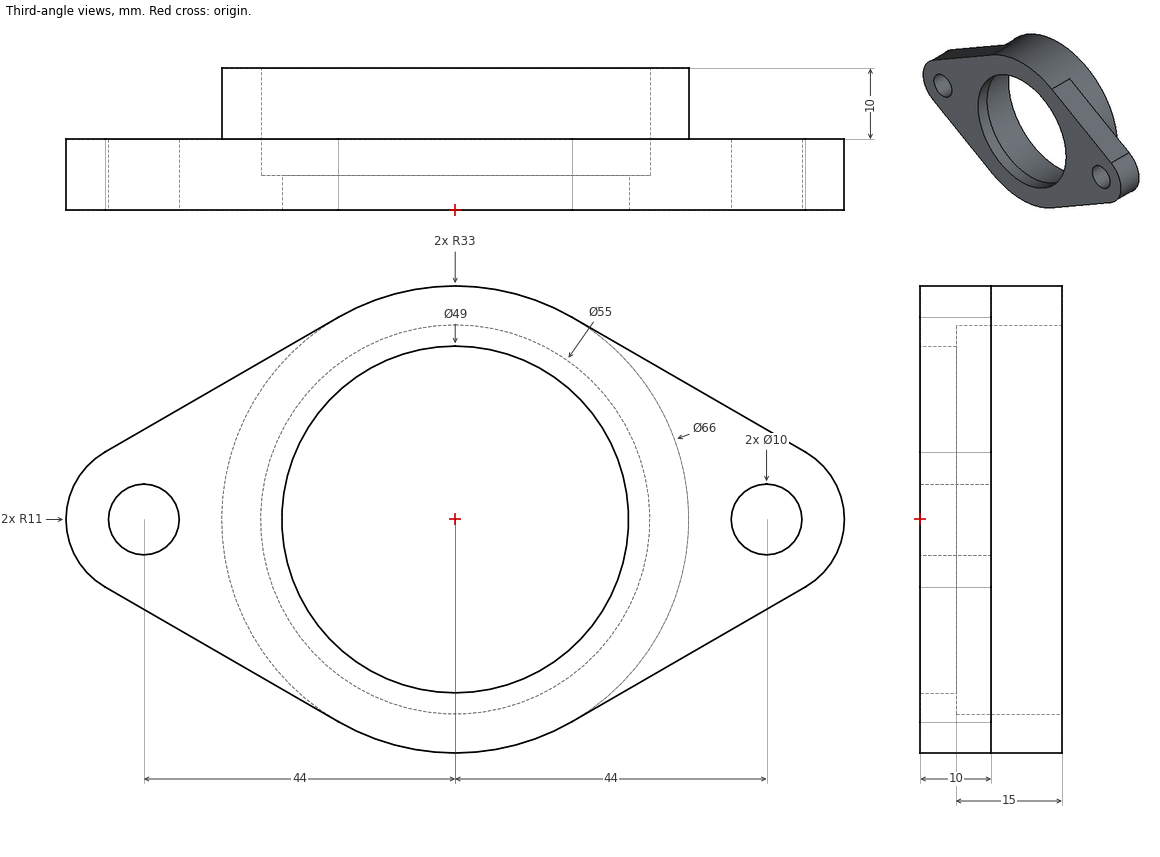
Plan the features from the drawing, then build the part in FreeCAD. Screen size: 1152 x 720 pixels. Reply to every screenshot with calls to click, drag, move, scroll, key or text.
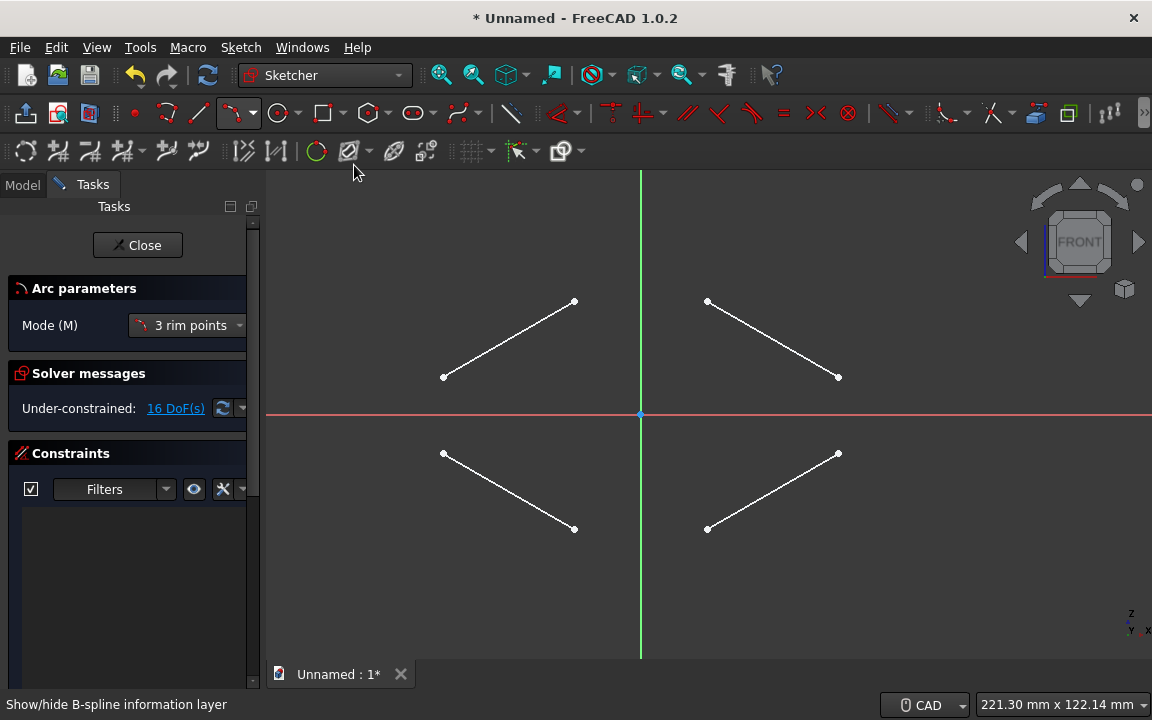
click(443, 454)
click(443, 377)
click(424, 397)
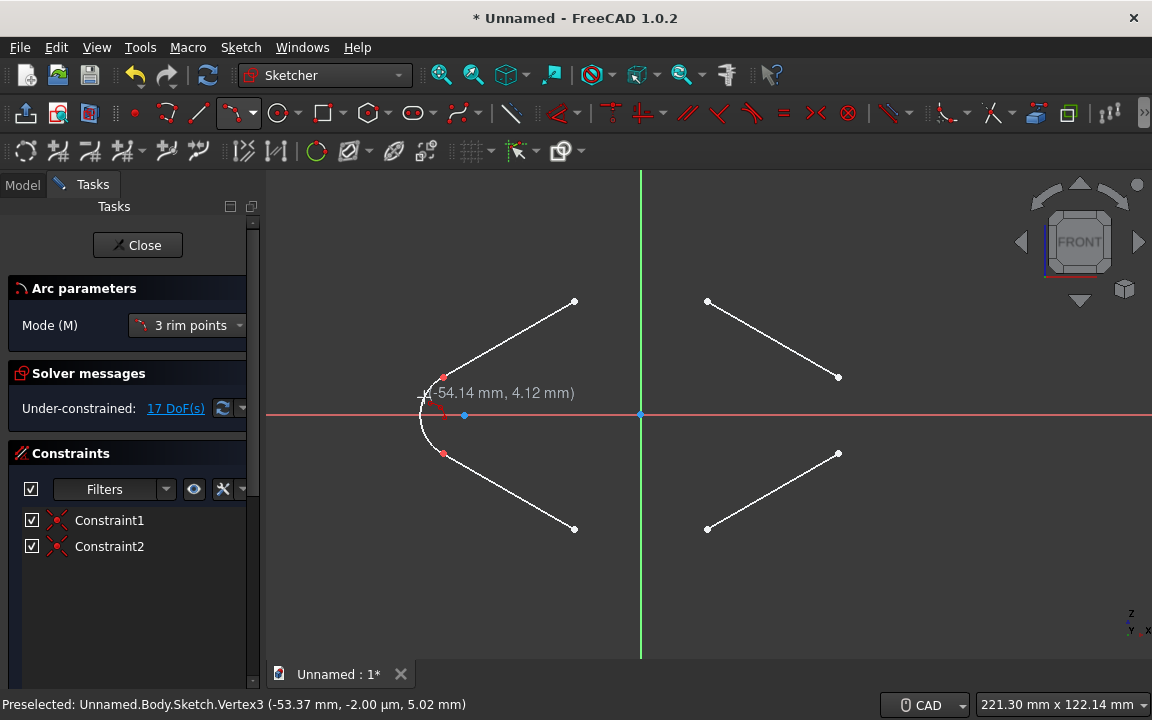
click(575, 301)
click(707, 301)
click(668, 285)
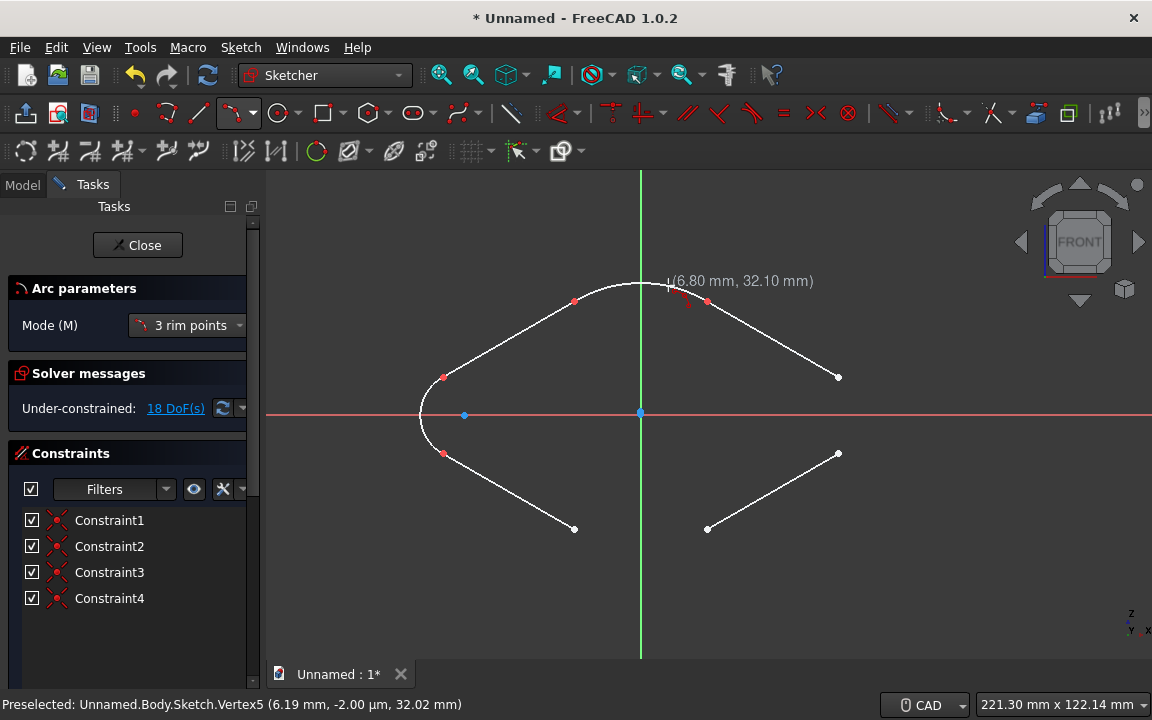
click(838, 377)
click(838, 454)
click(857, 432)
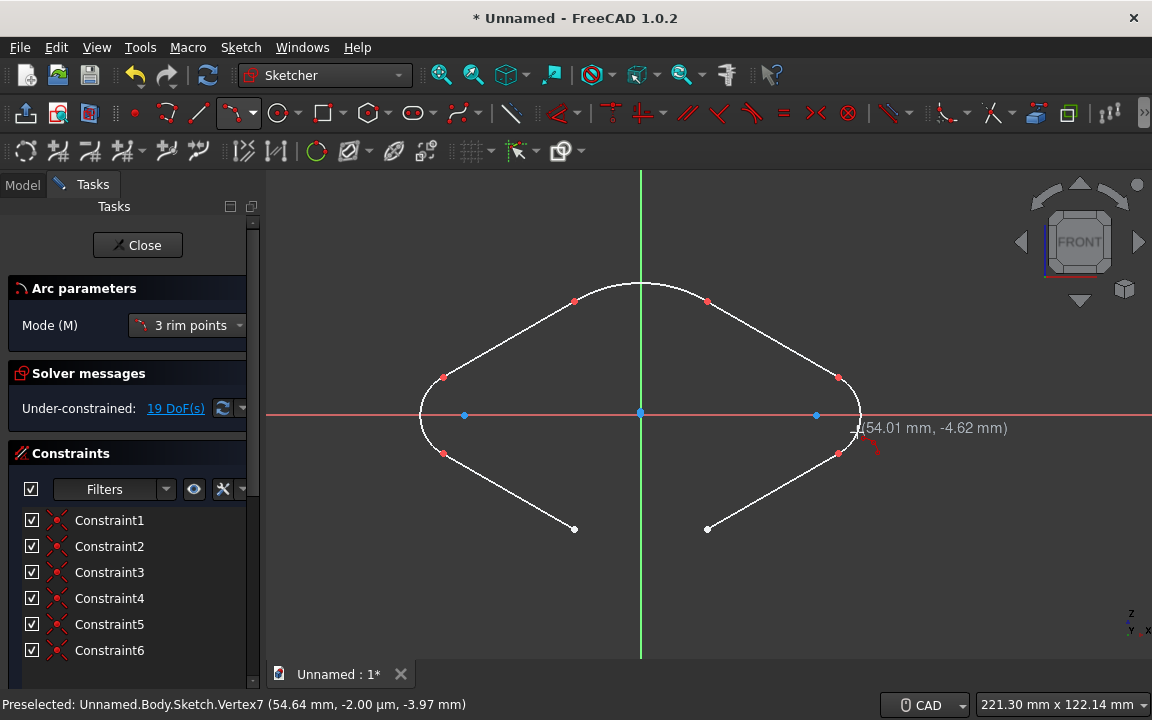
click(707, 530)
click(575, 530)
click(613, 544)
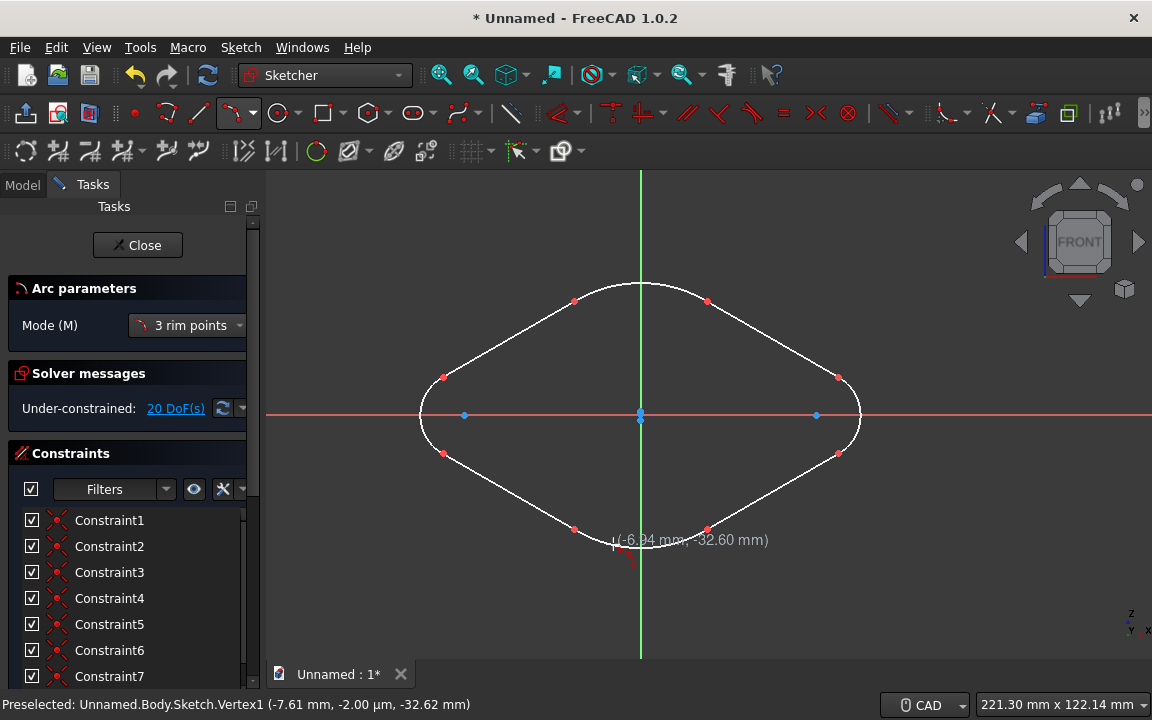
click(278, 114)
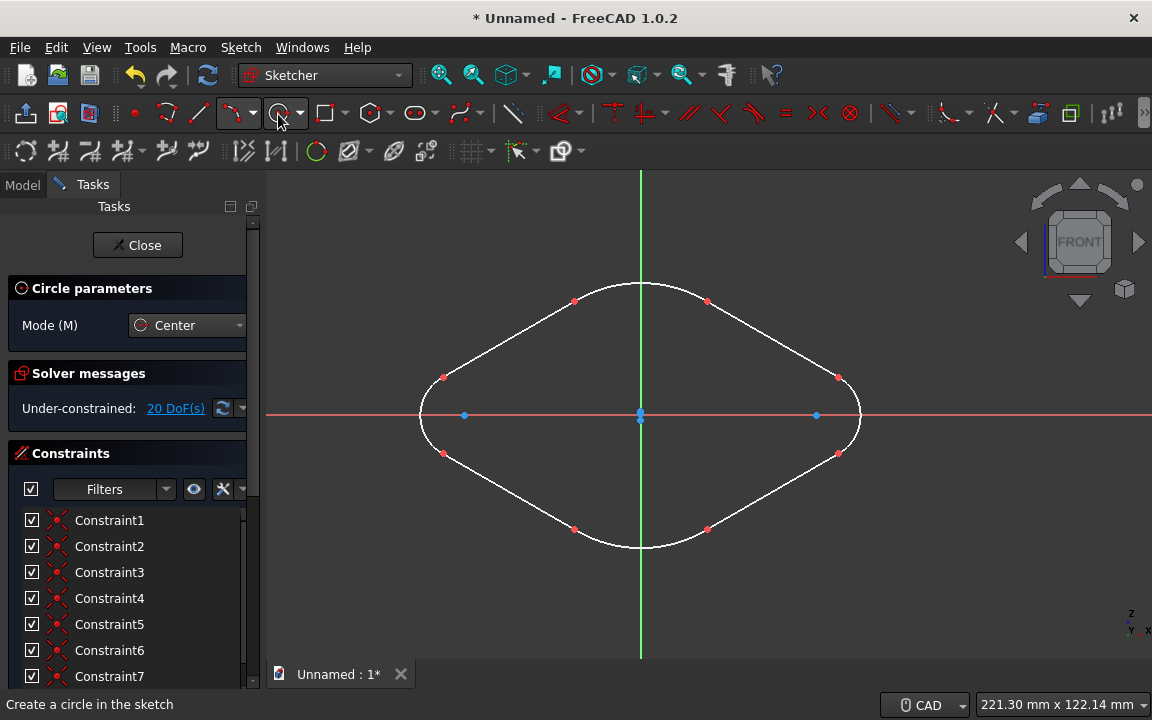
click(817, 414)
move(831, 400)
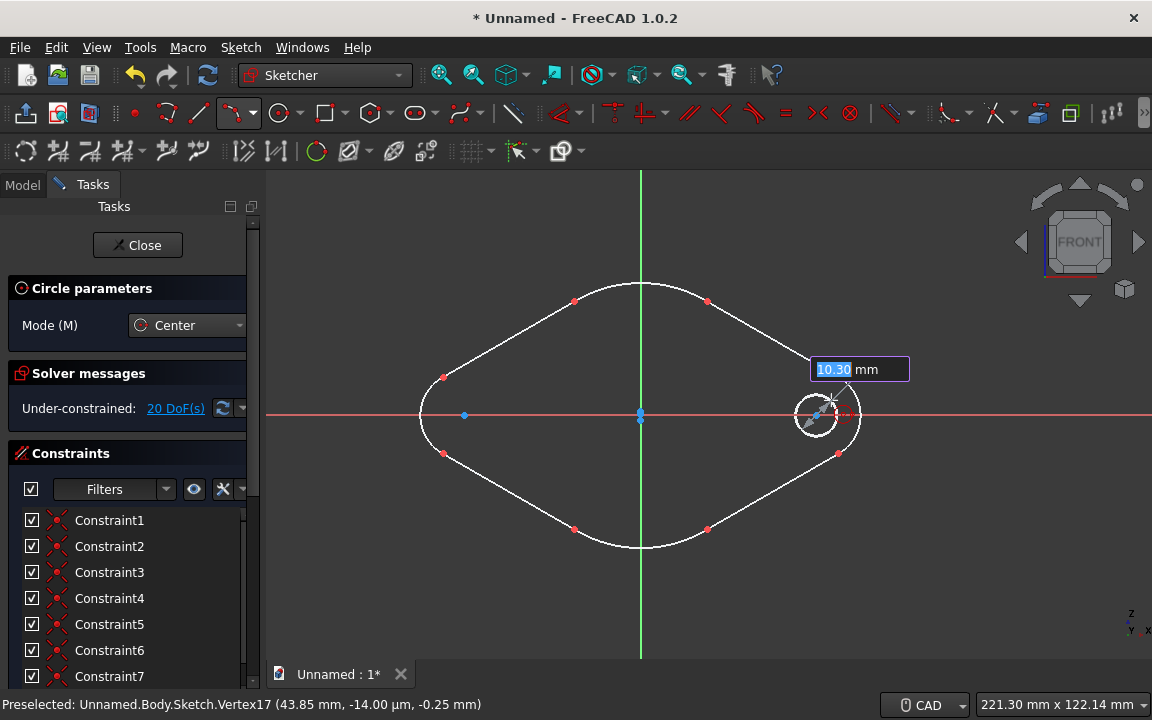
text(10)
key(Return)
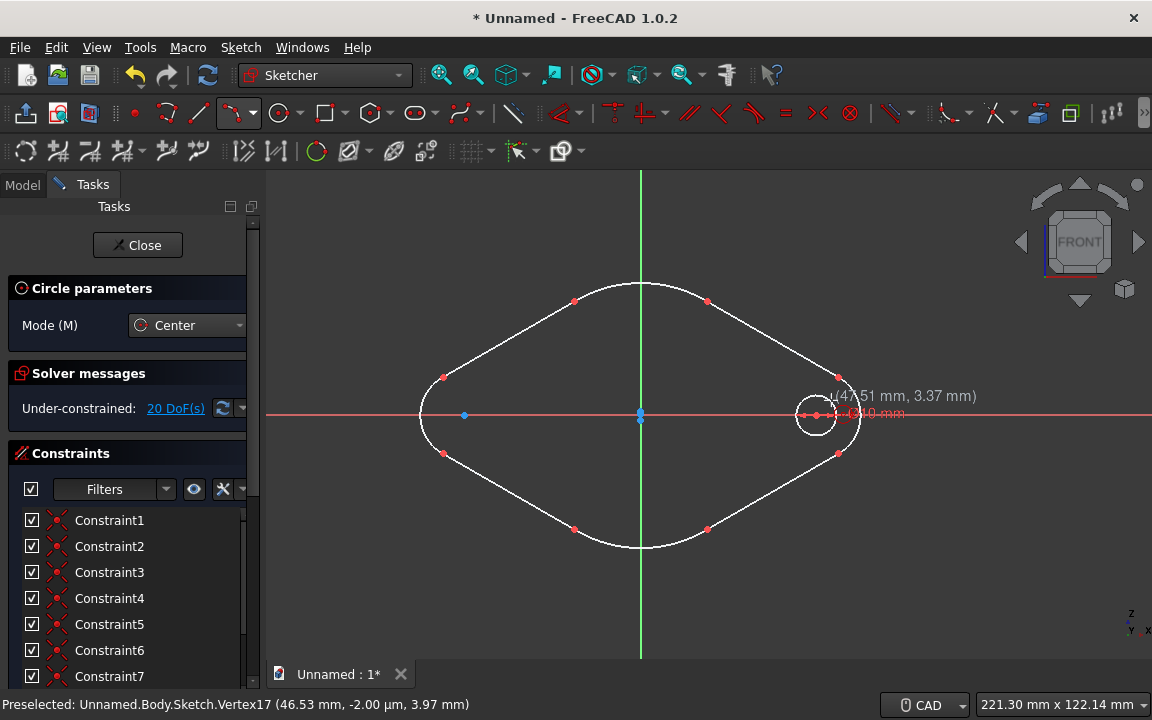
click(465, 414)
move(479, 400)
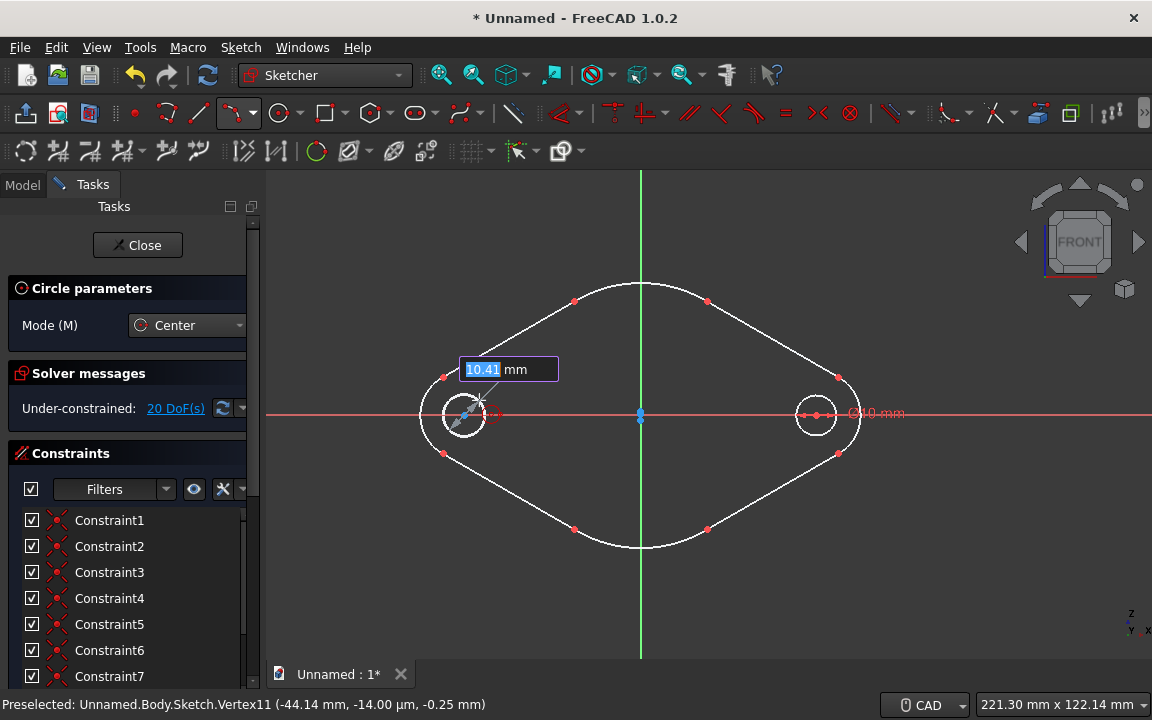
text(10)
key(Return)
key(Escape)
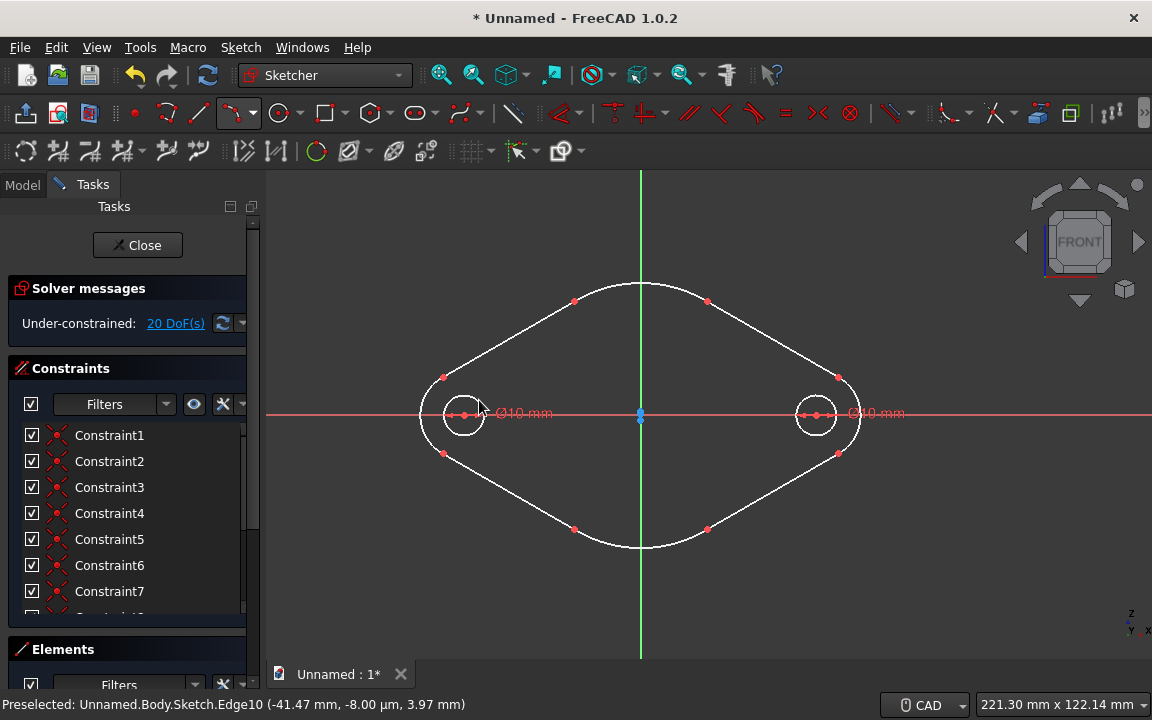
click(535, 507)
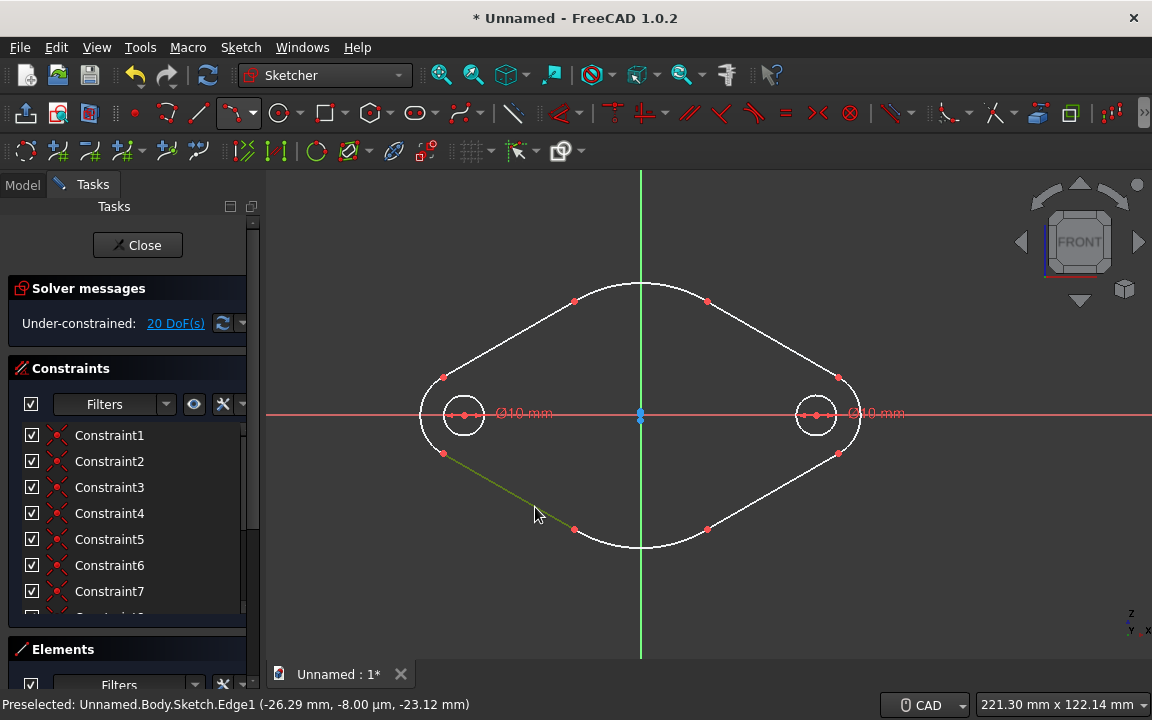
click(424, 397)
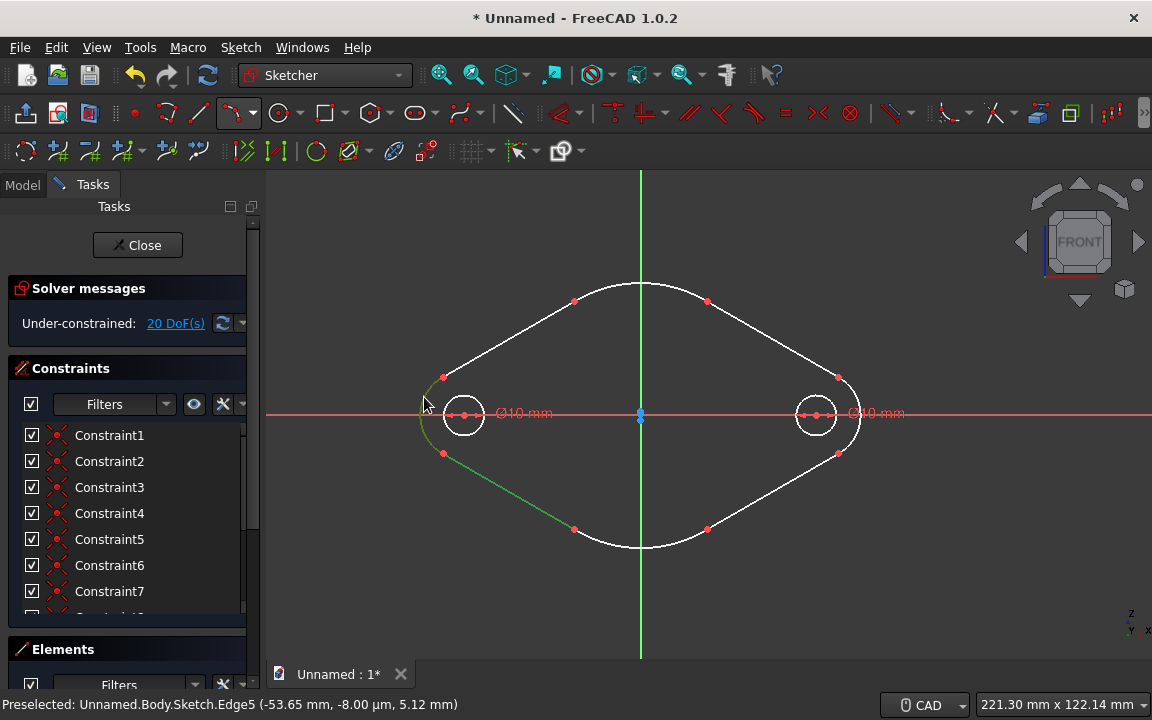
click(754, 114)